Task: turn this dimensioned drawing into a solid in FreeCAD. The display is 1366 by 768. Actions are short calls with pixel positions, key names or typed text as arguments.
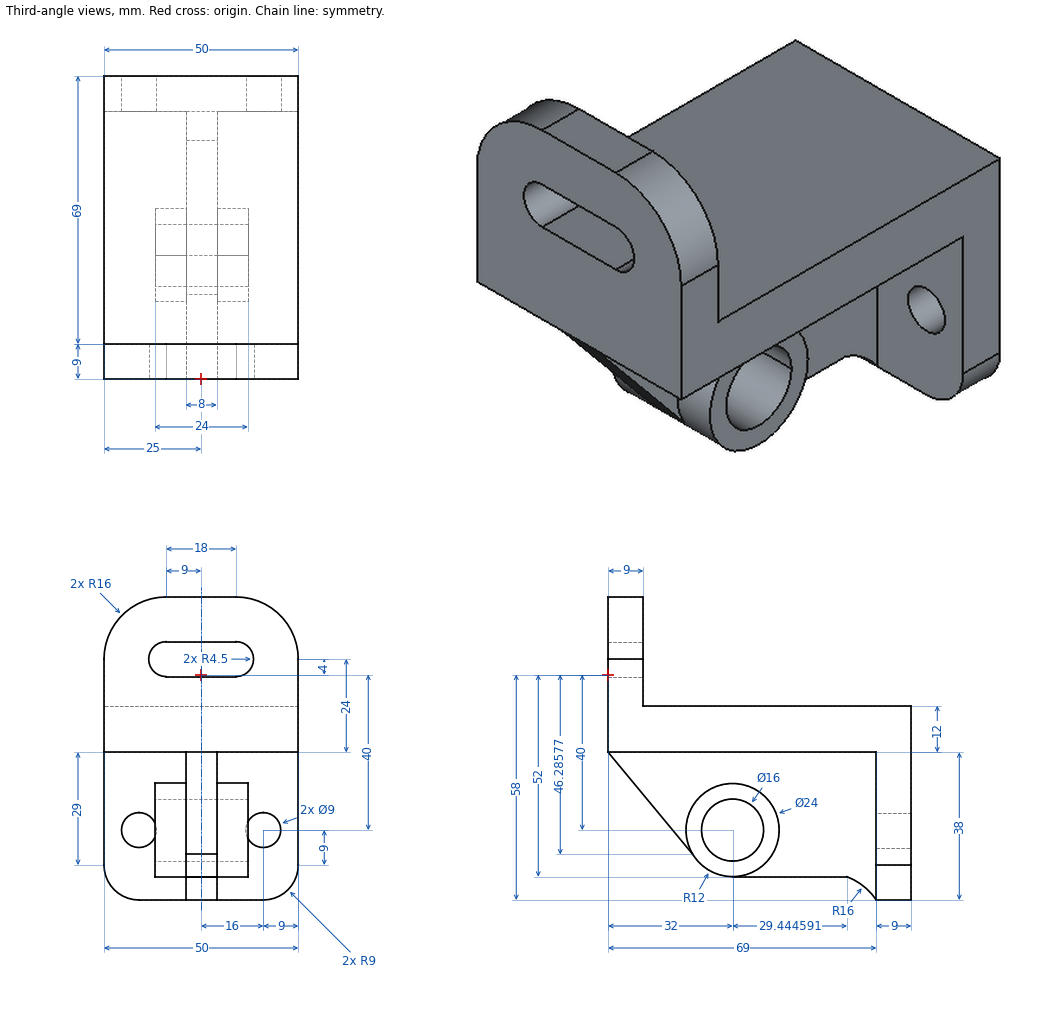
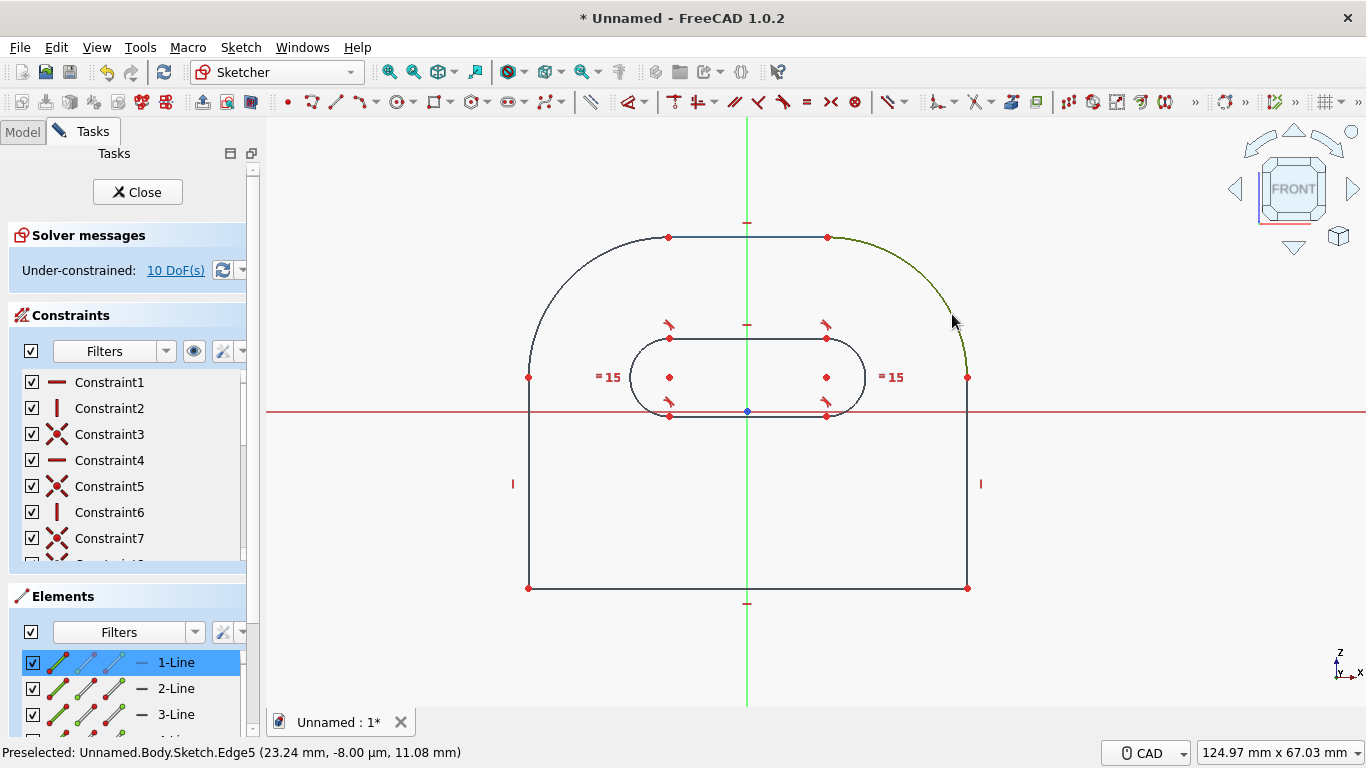
key(t)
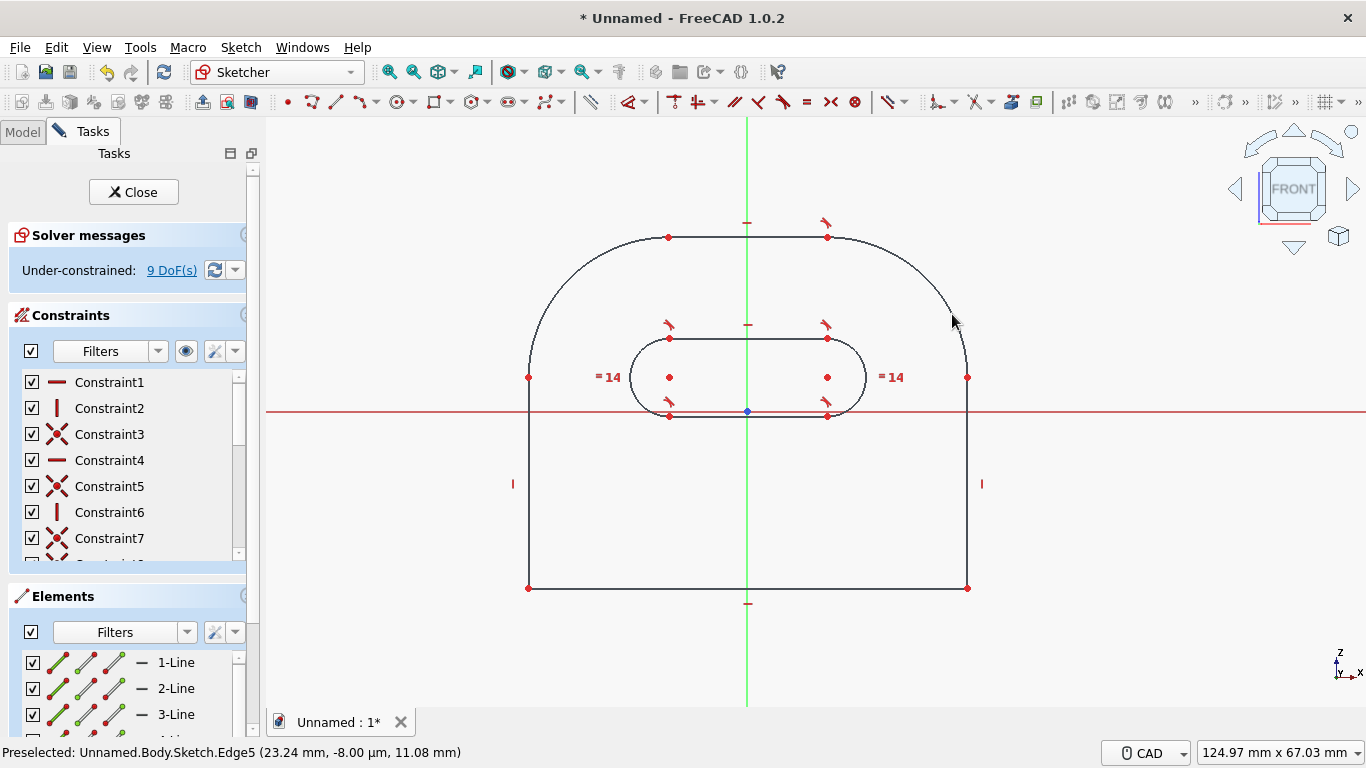
click(716, 237)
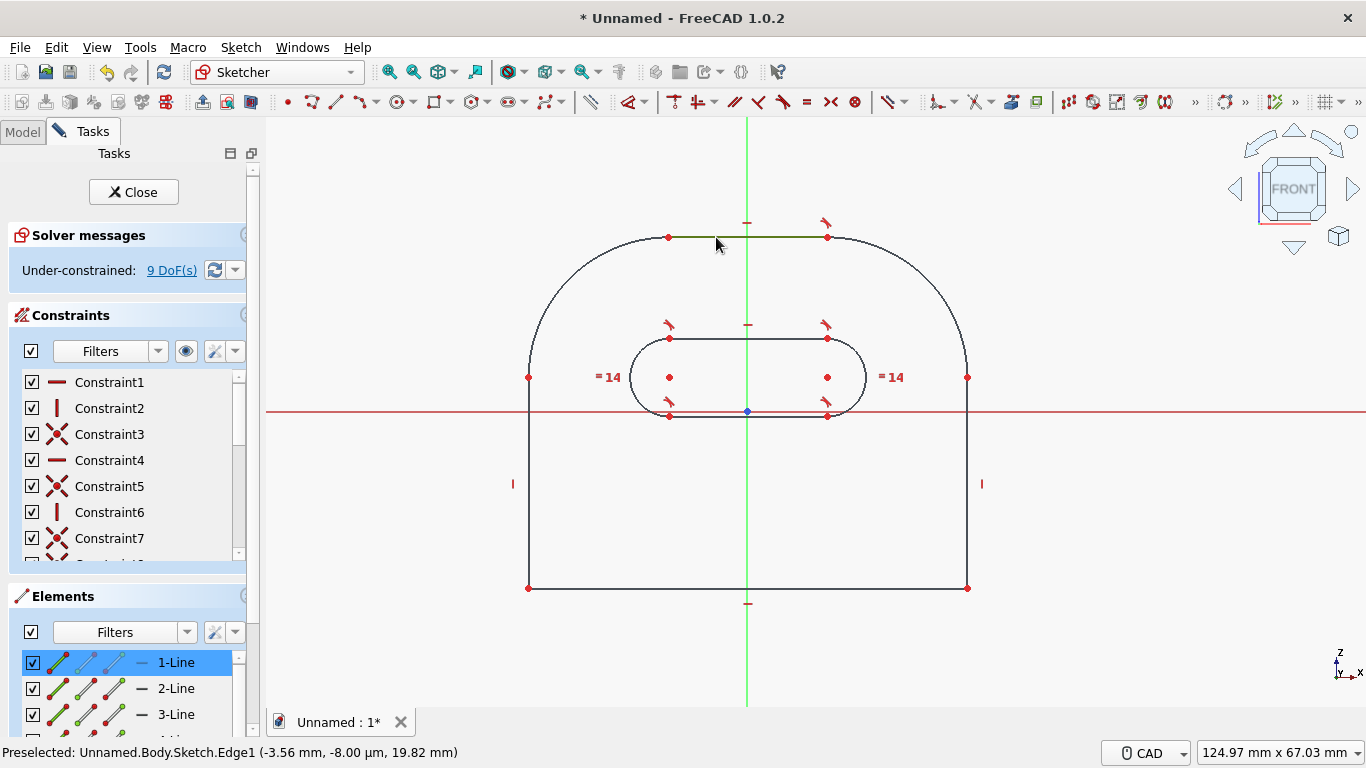
click(605, 253)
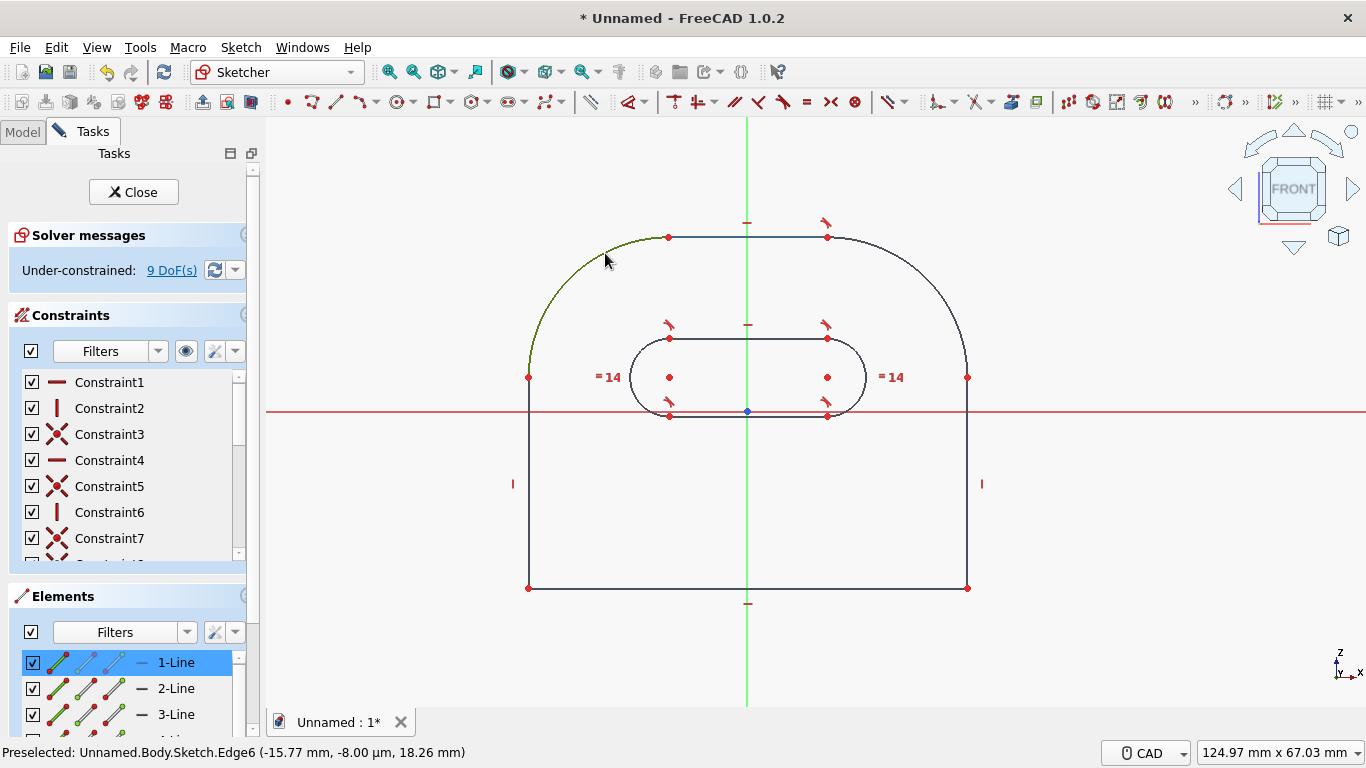
key(t)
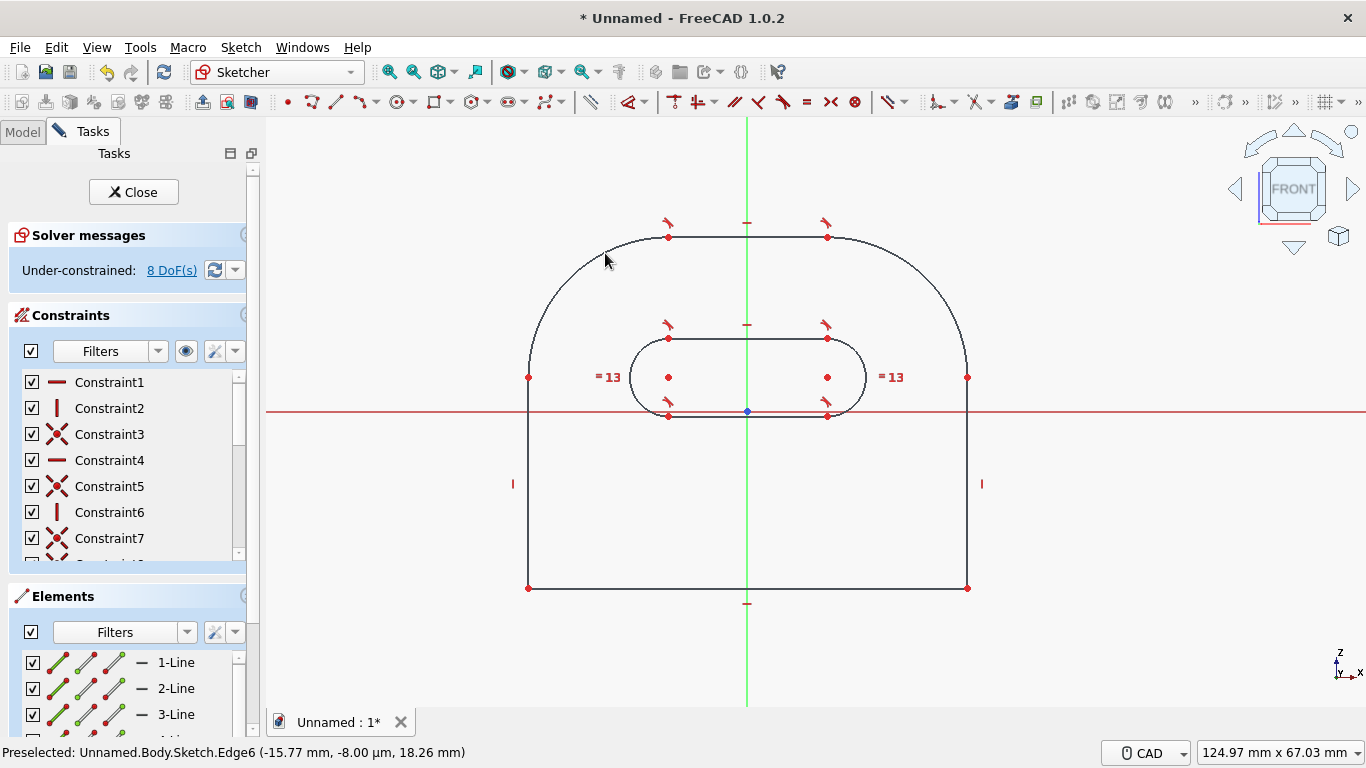
click(967, 441)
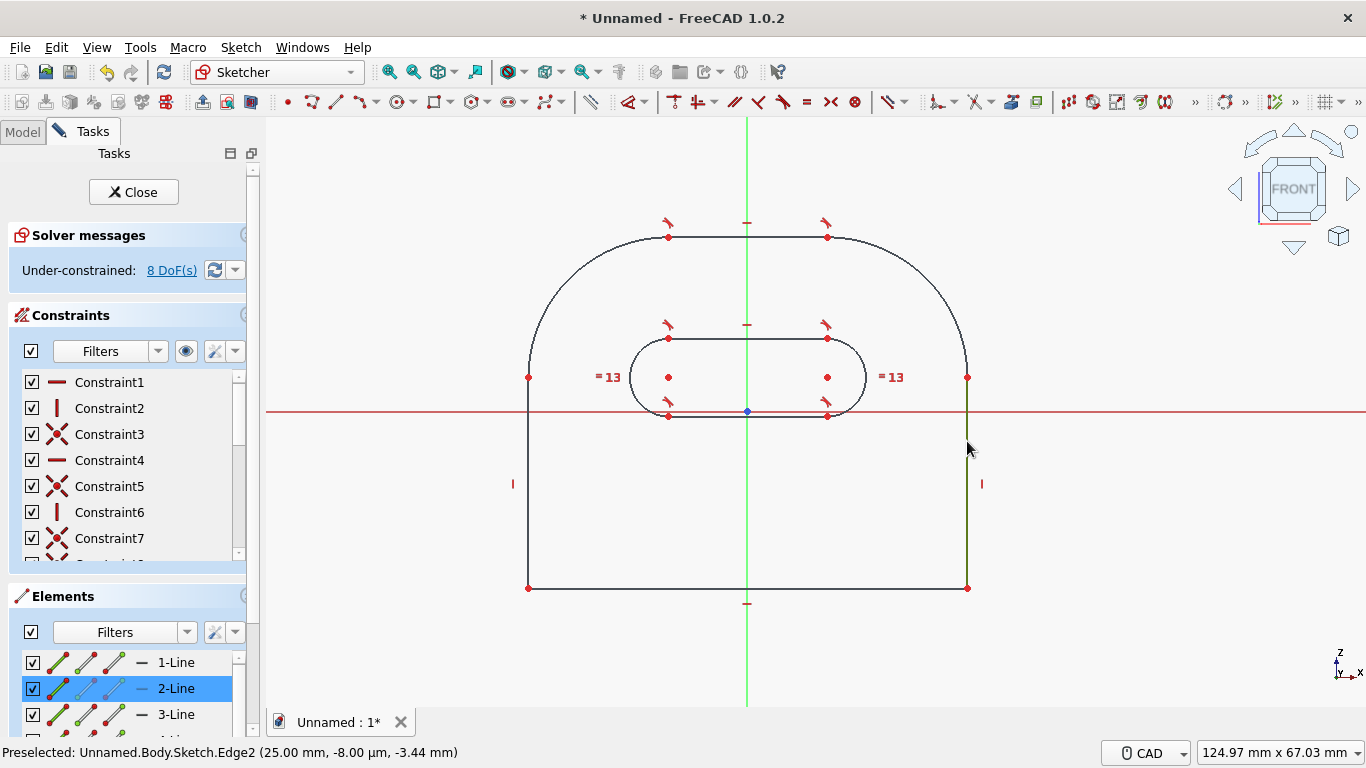
click(952, 314)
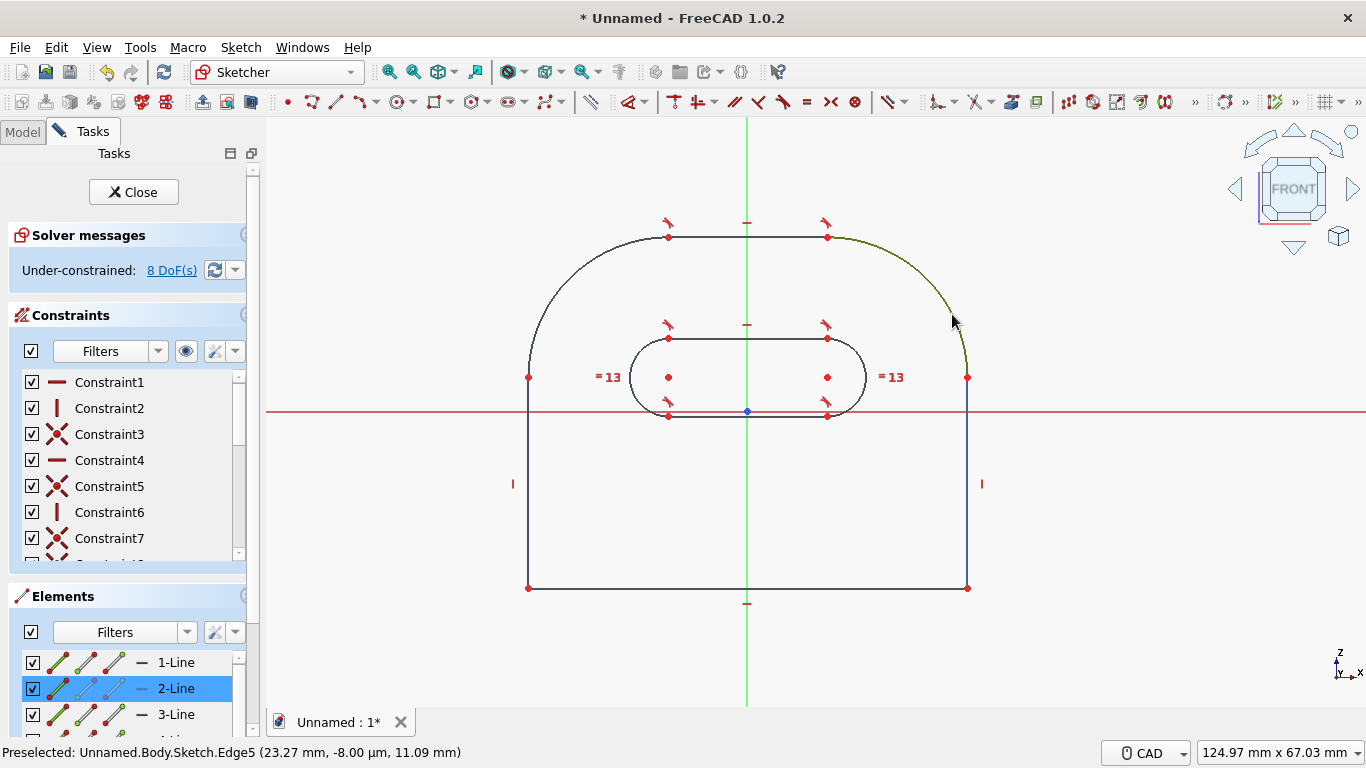
click(784, 102)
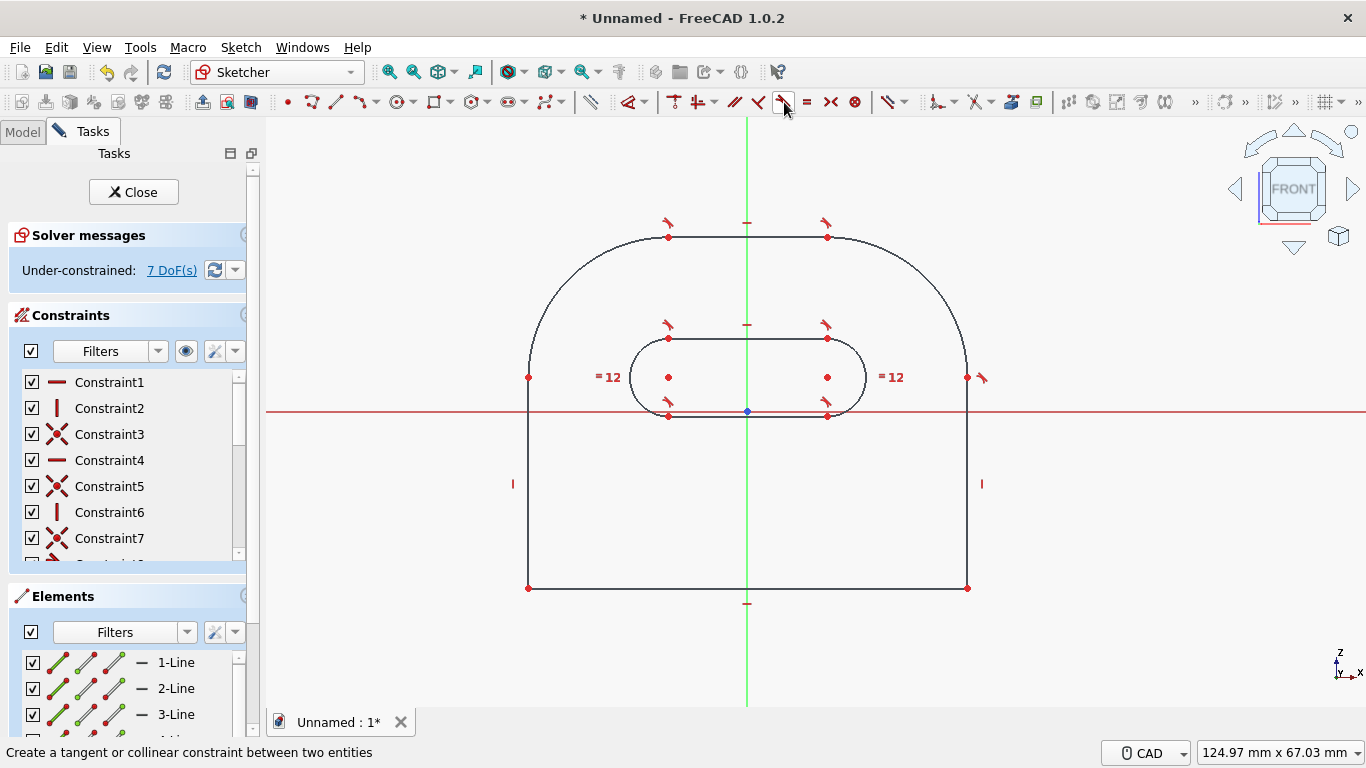
click(528, 526)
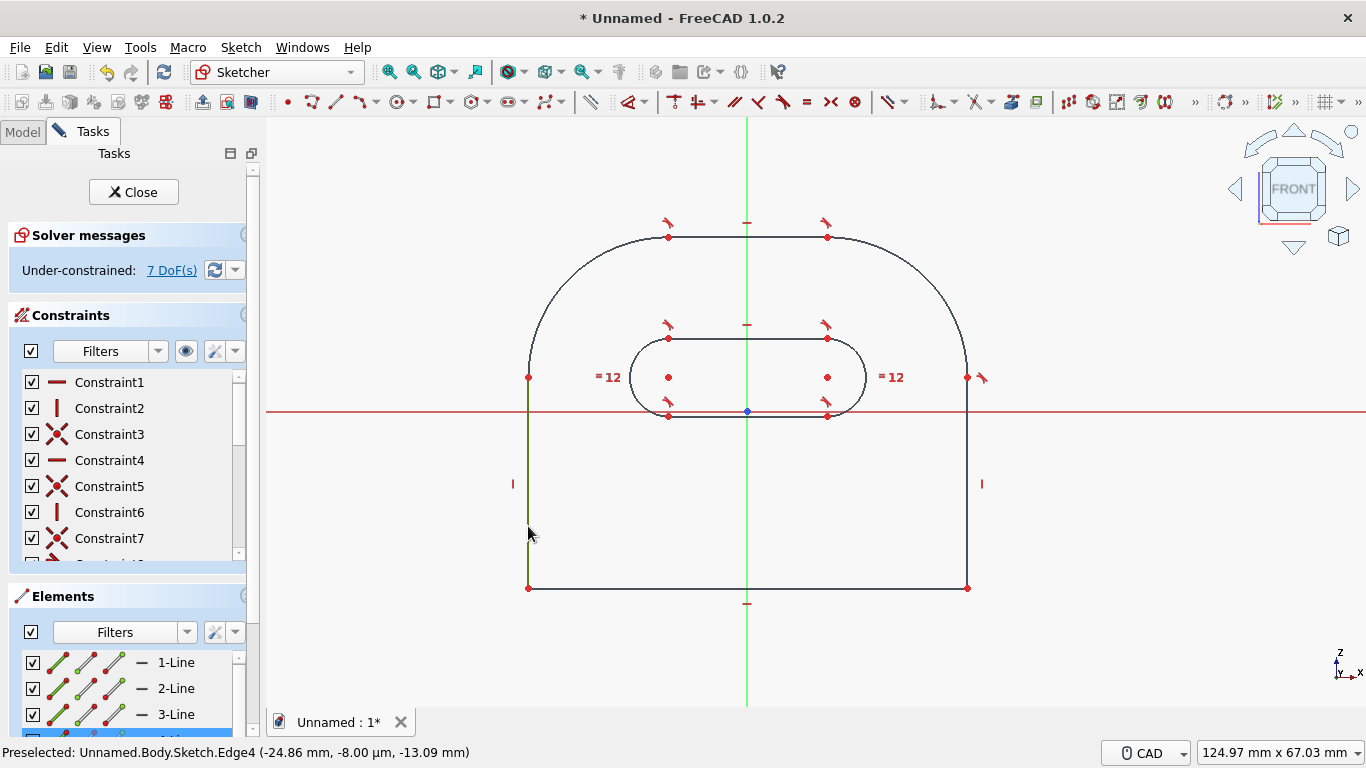
click(605, 253)